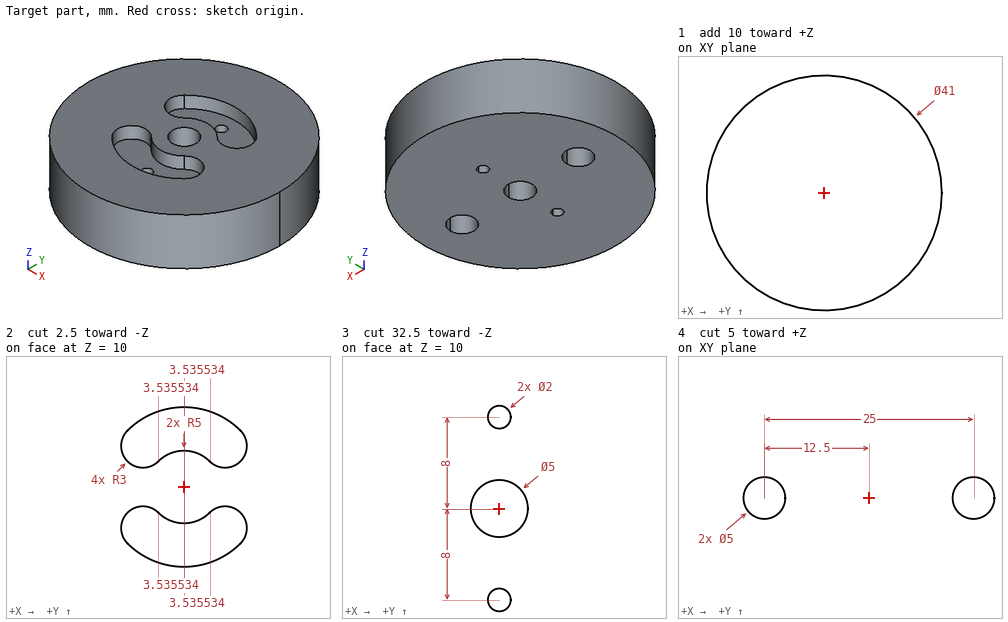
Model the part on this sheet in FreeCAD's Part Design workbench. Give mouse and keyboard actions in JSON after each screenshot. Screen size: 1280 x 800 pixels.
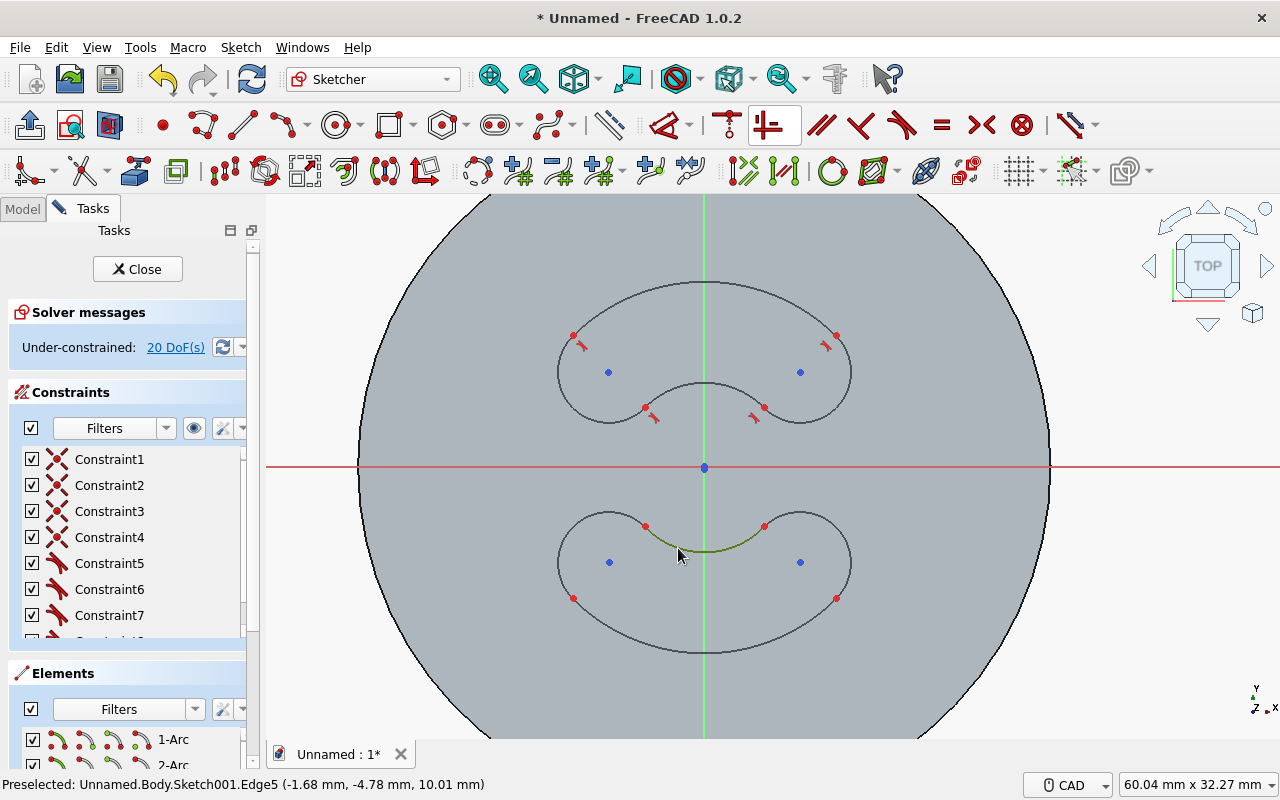
{"action": "left_click", "coordinate": [601, 513]}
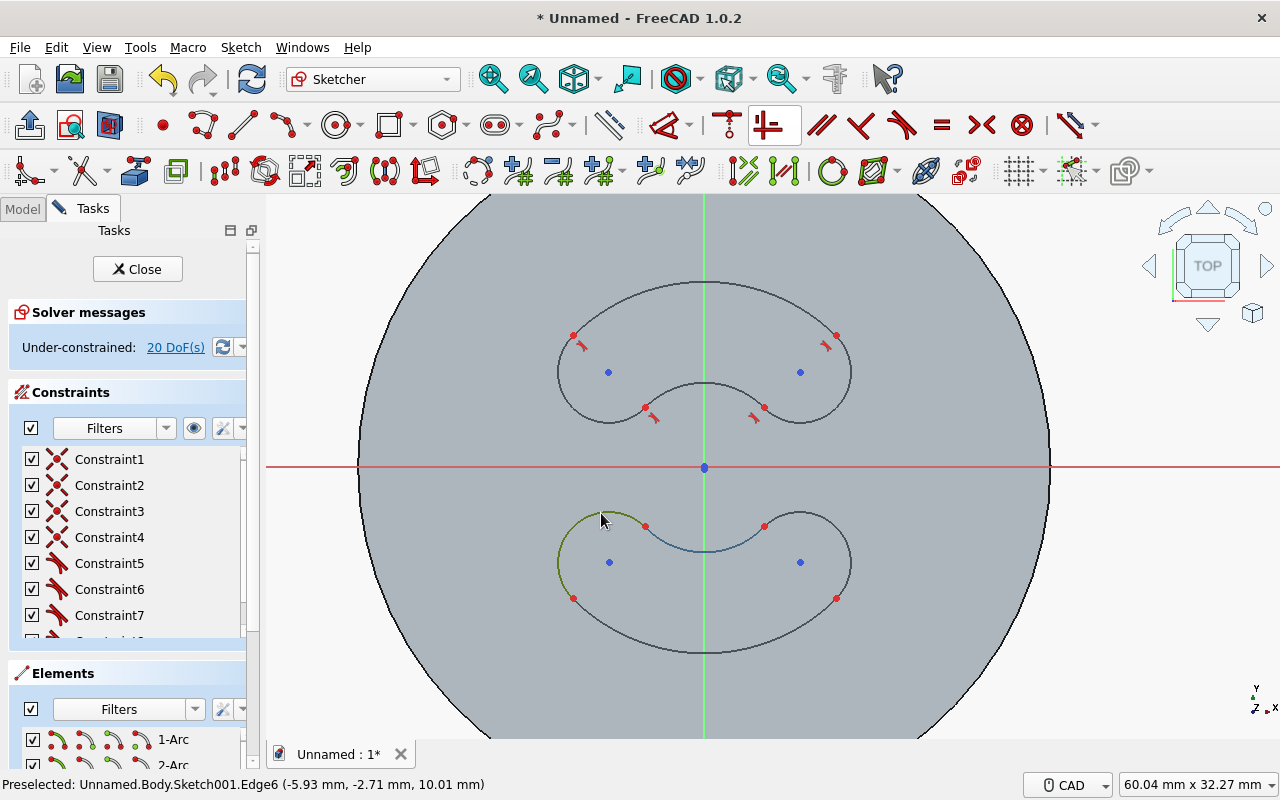
{"action": "key", "text": "t"}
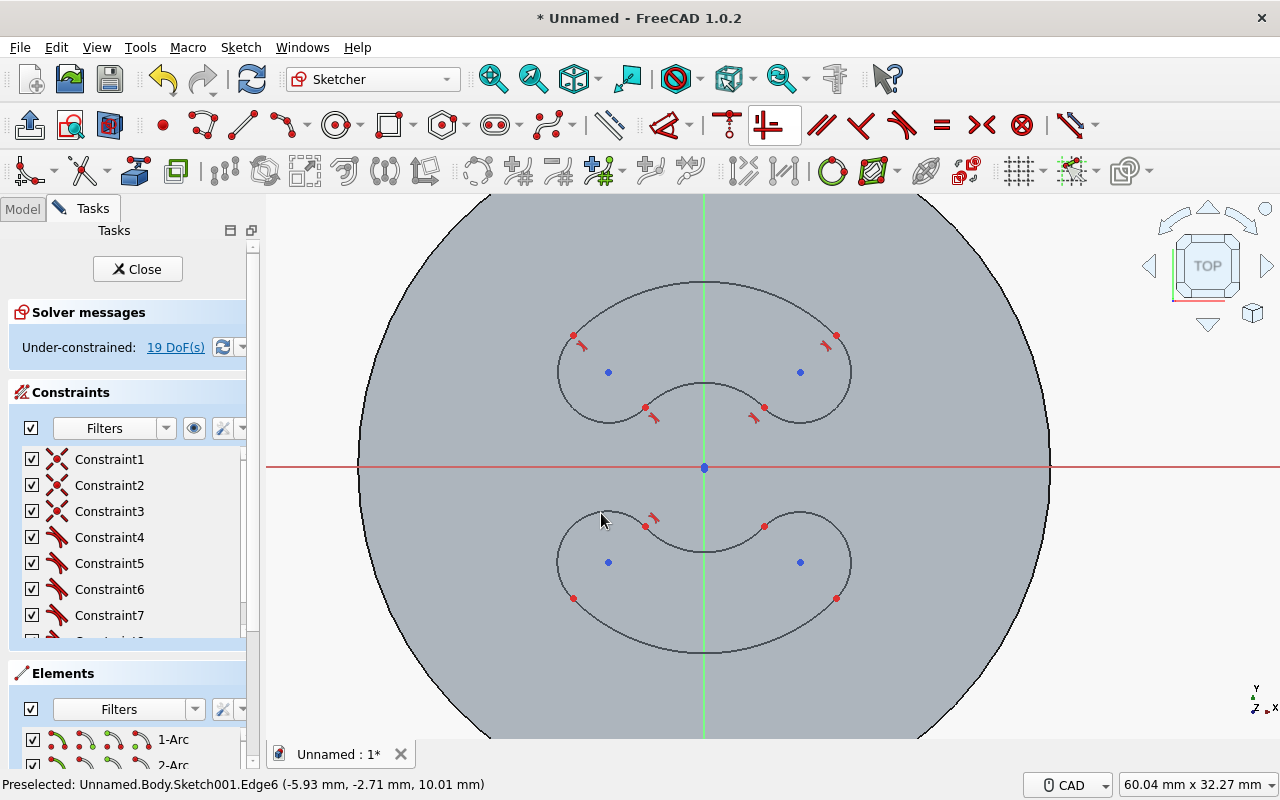
{"action": "left_click", "coordinate": [678, 548]}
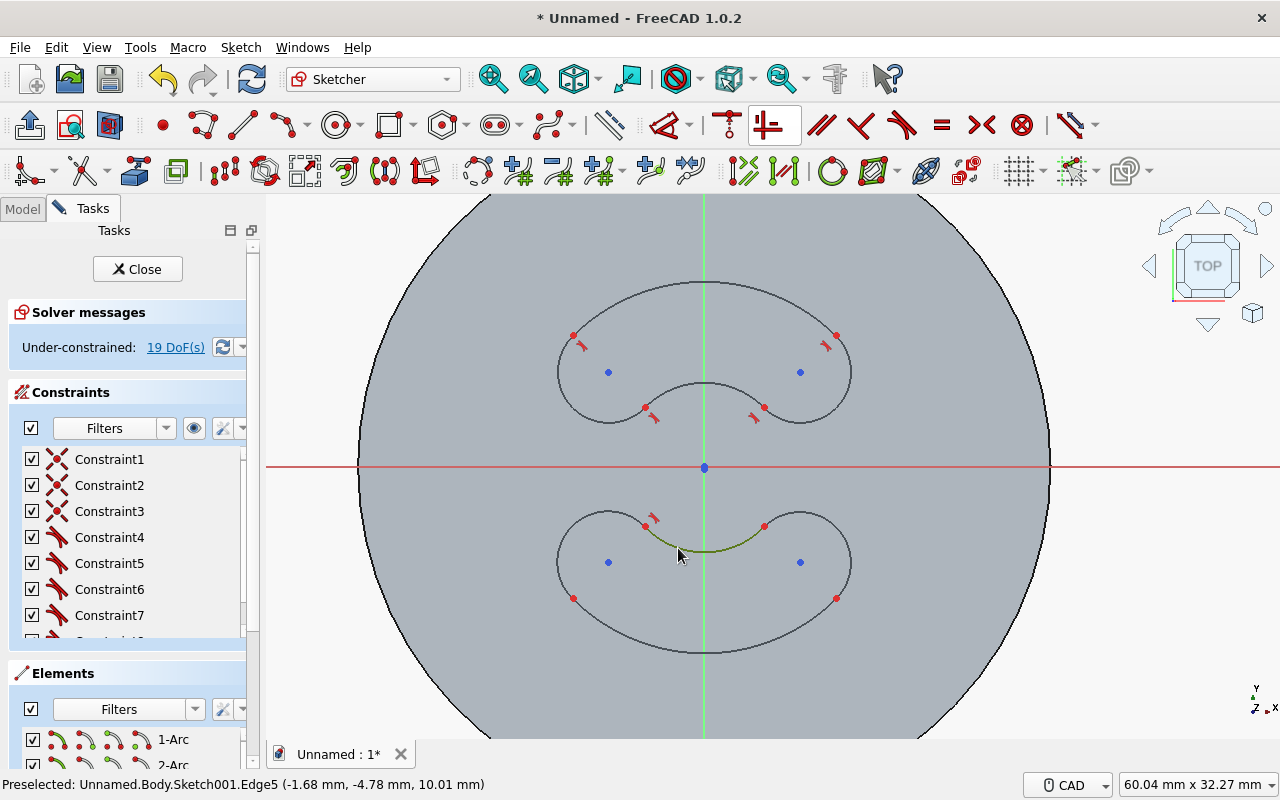
{"action": "left_click", "coordinate": [850, 555]}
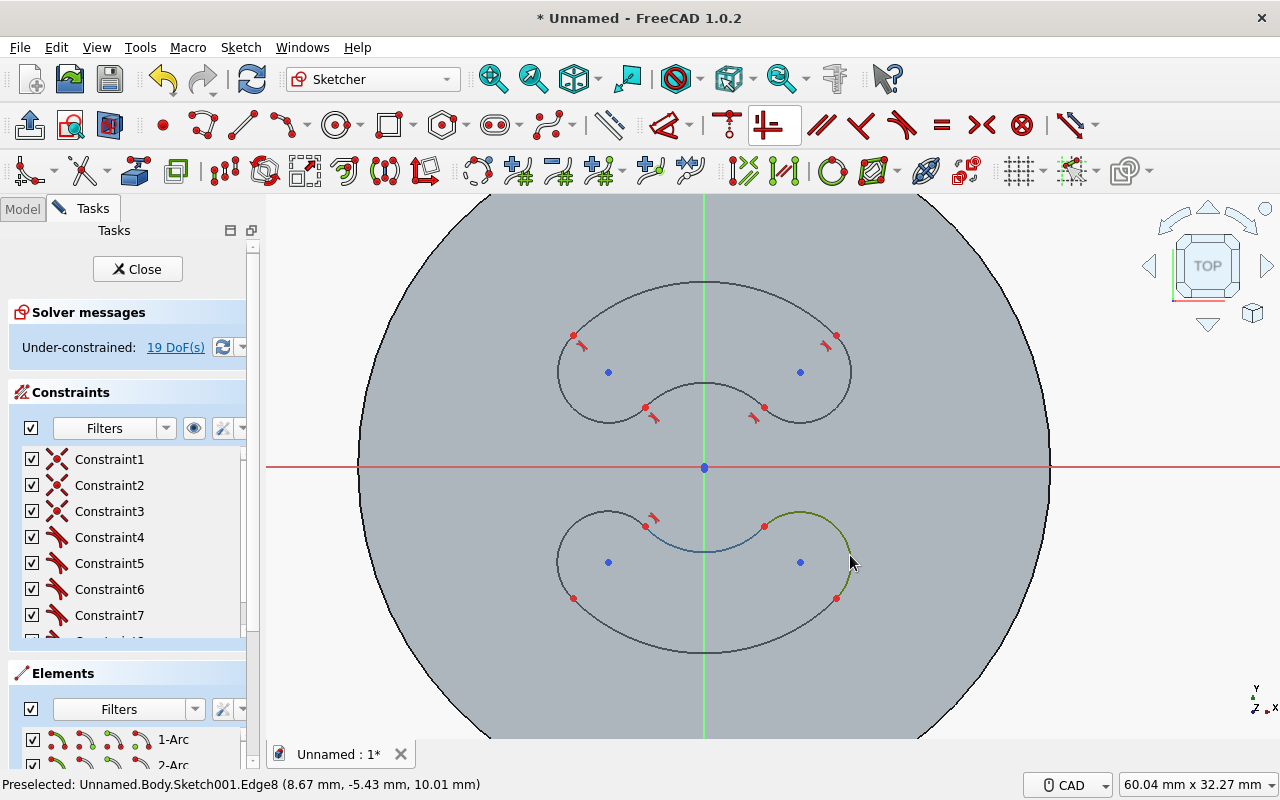
{"action": "key", "text": "t"}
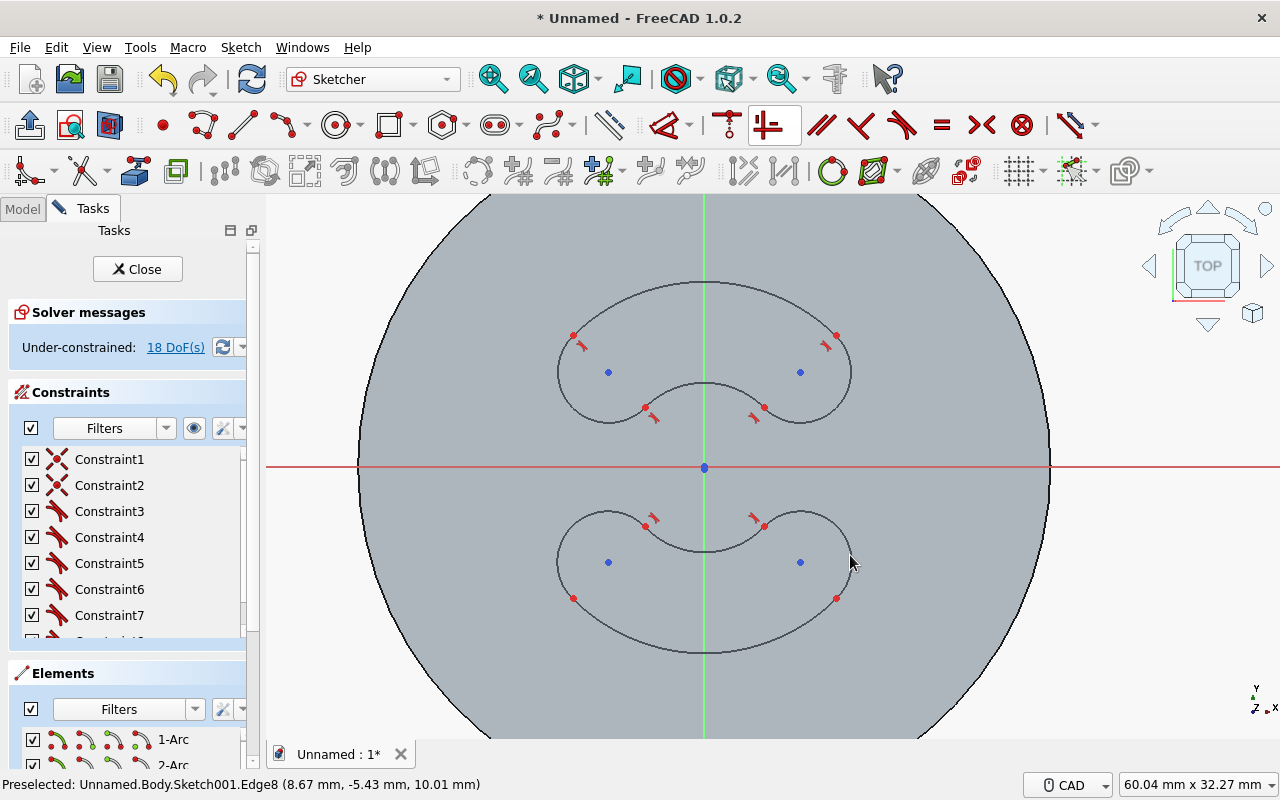
{"action": "left_click", "coordinate": [601, 512]}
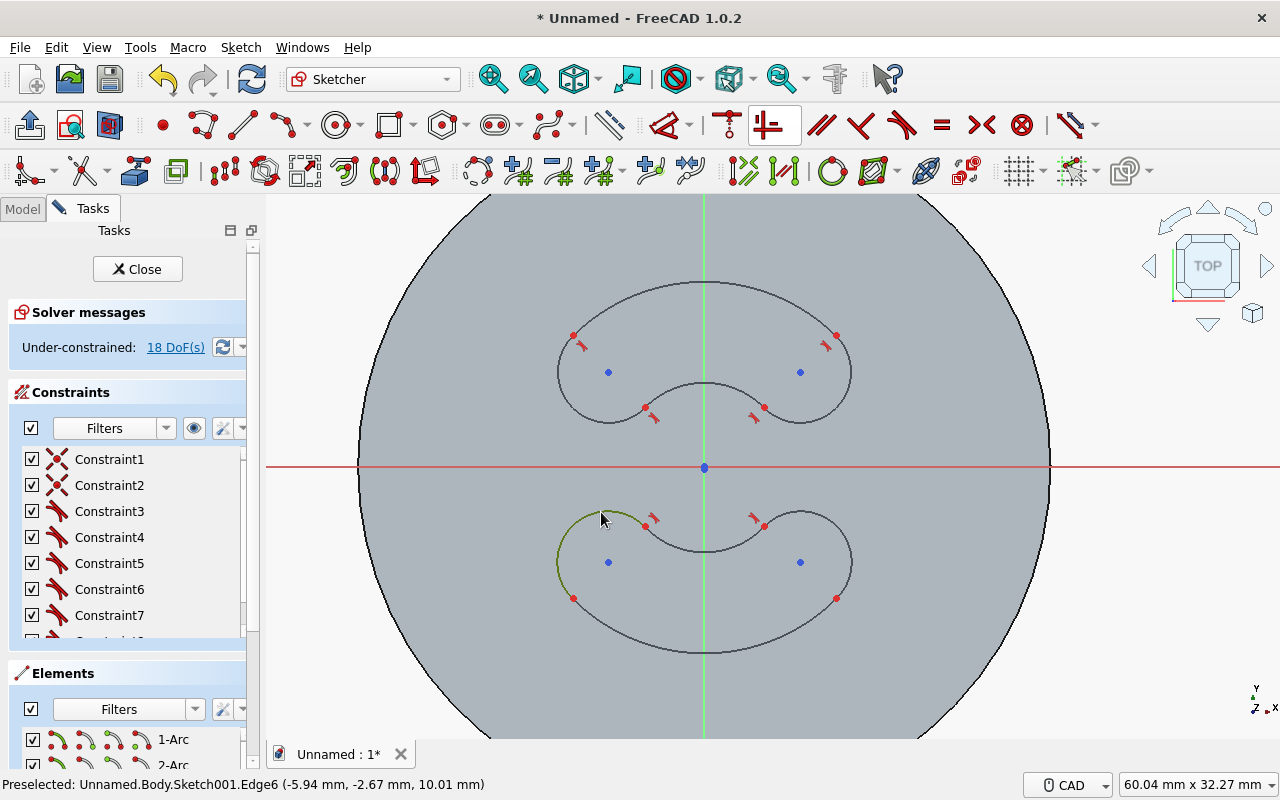
{"action": "left_click", "coordinate": [647, 644]}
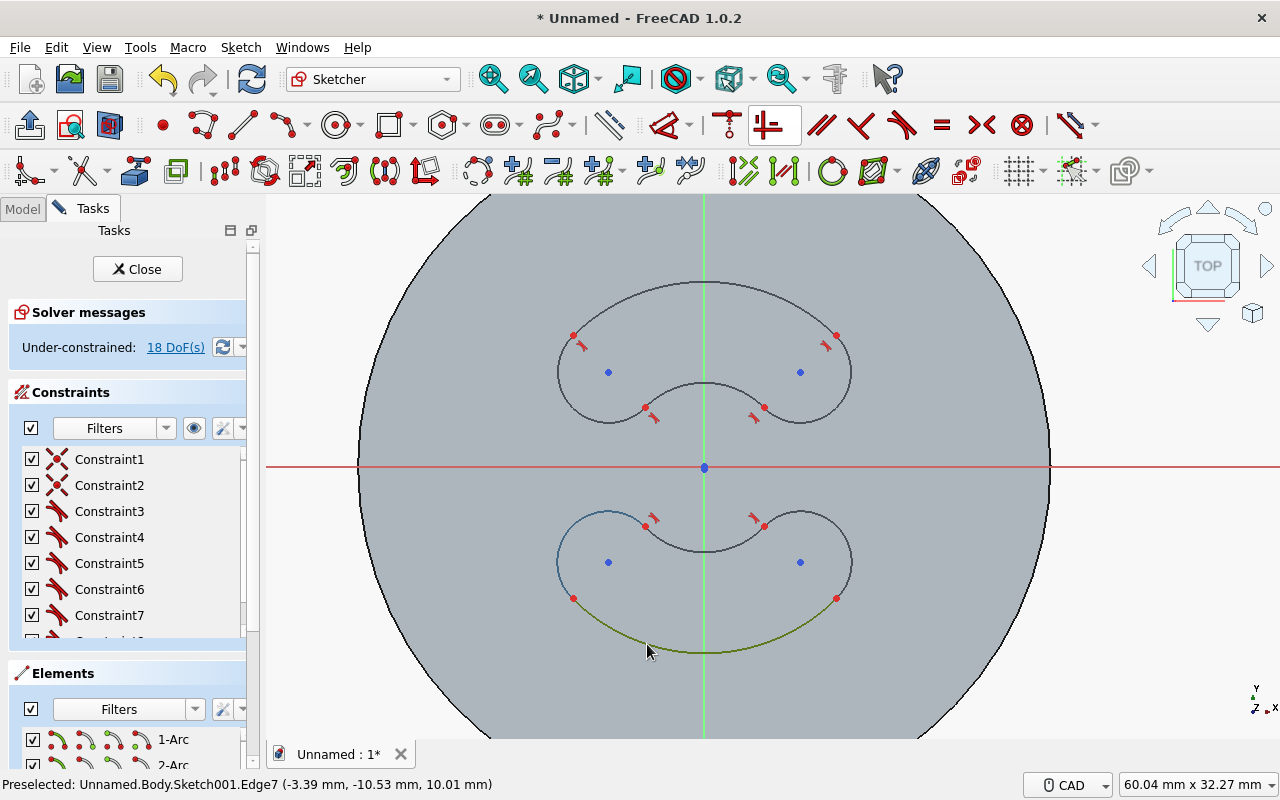
{"action": "key", "text": "t"}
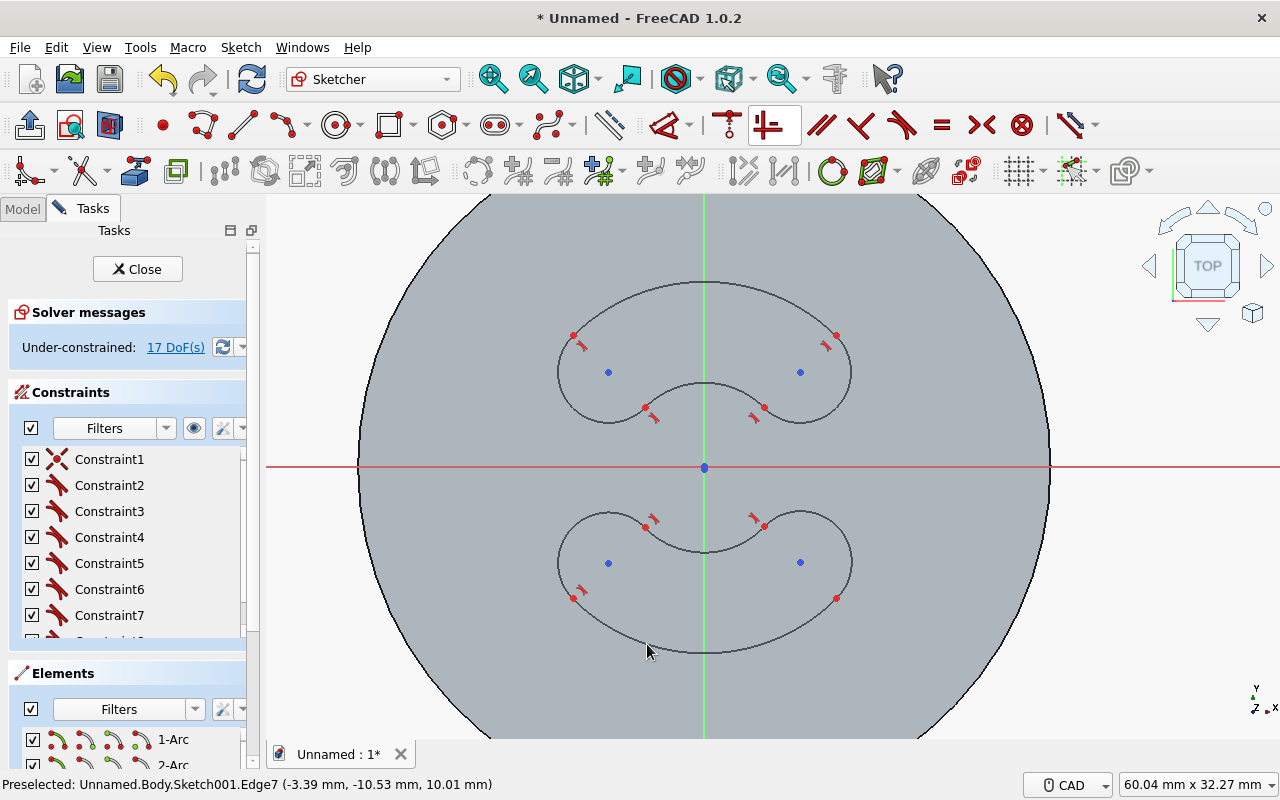
{"action": "left_click", "coordinate": [647, 644]}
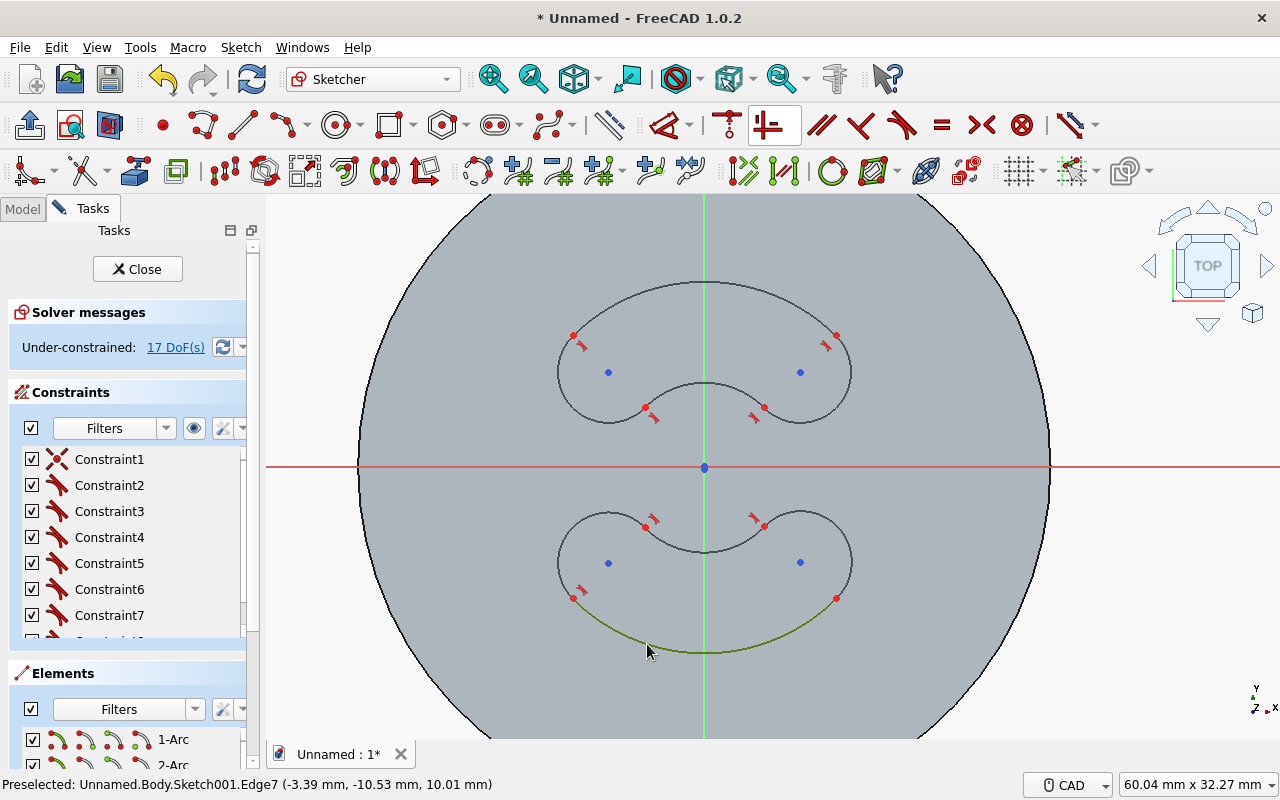
{"action": "left_click", "coordinate": [851, 555]}